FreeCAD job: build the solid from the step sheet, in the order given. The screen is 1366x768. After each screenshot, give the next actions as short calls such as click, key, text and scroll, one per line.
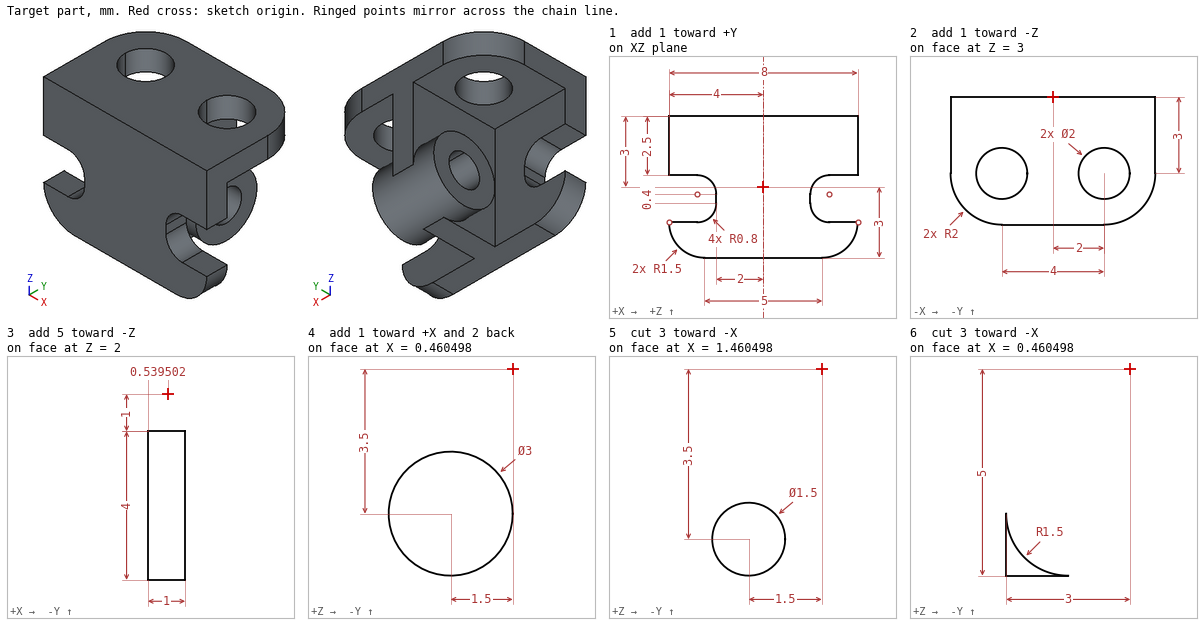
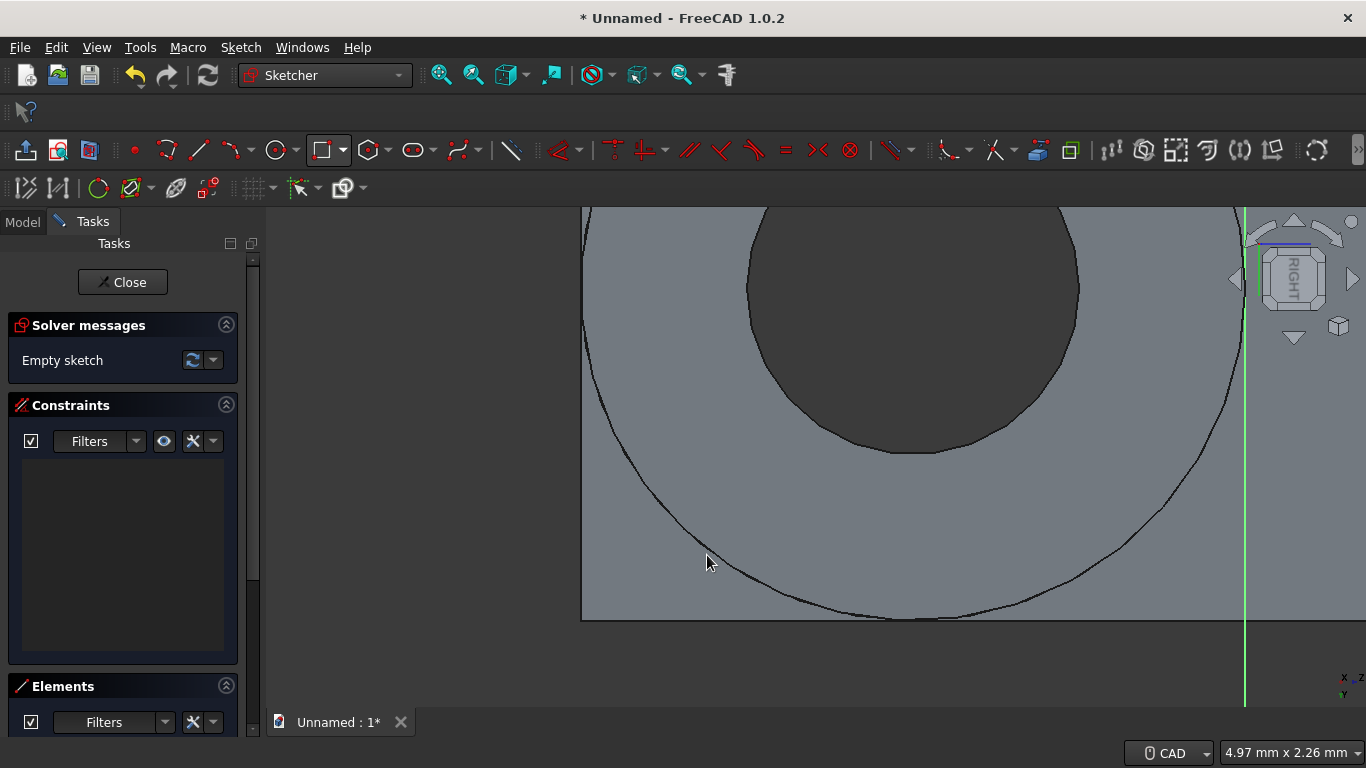
click(168, 150)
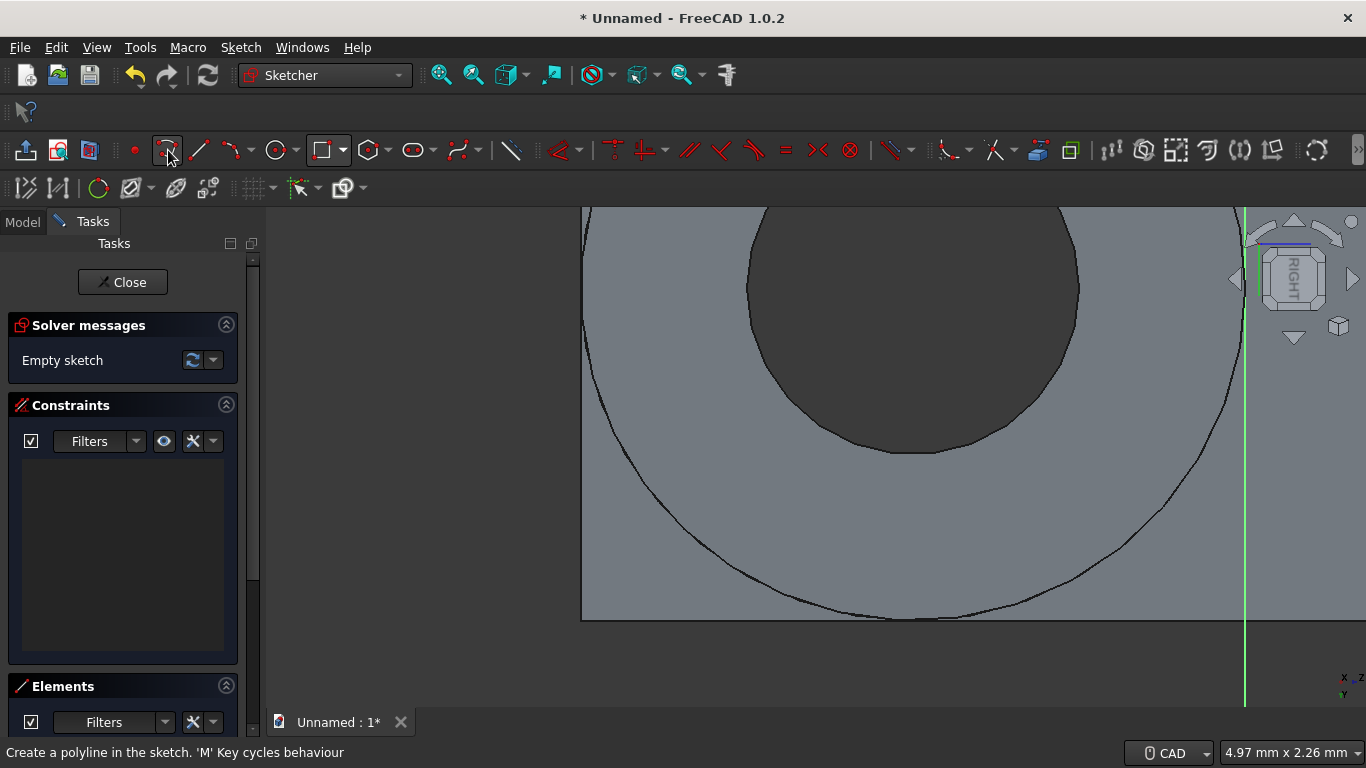
click(581, 288)
click(581, 621)
click(913, 621)
right_click(913, 621)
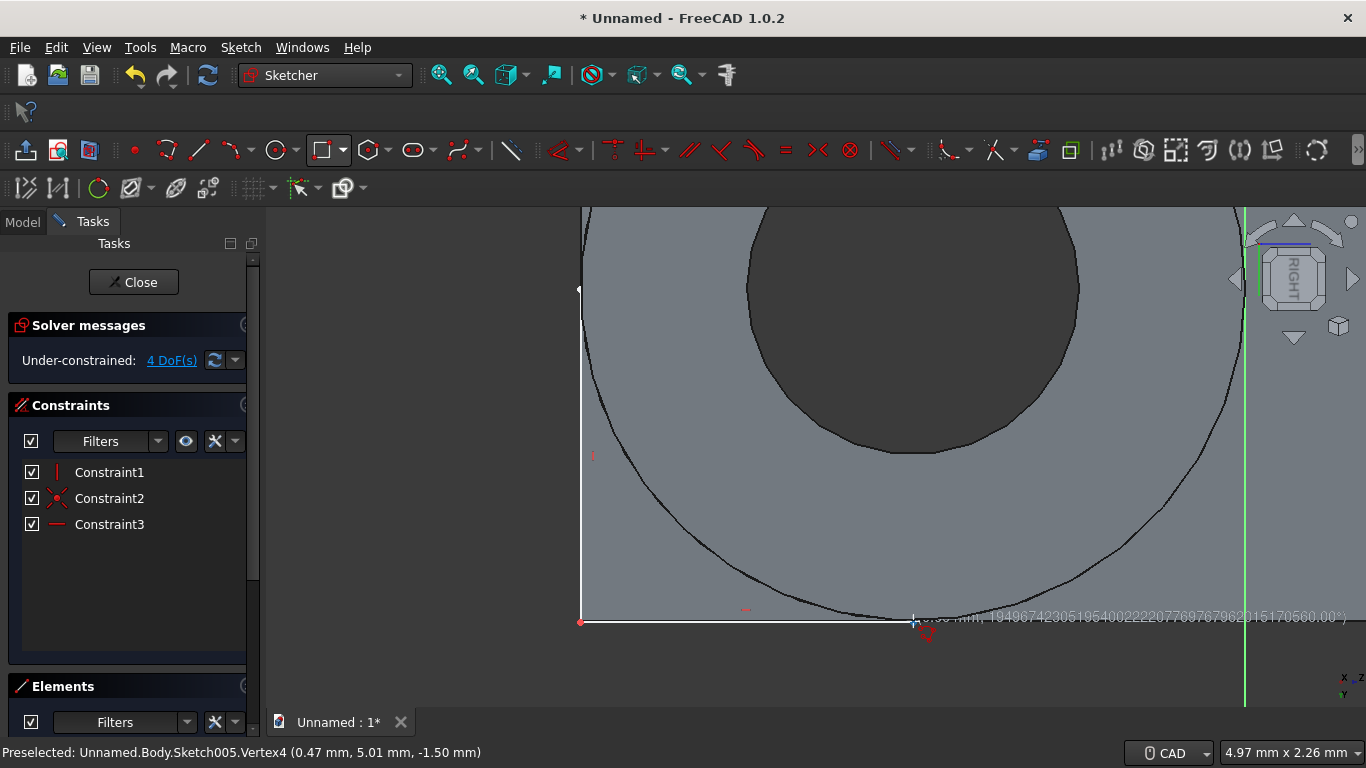
click(232, 150)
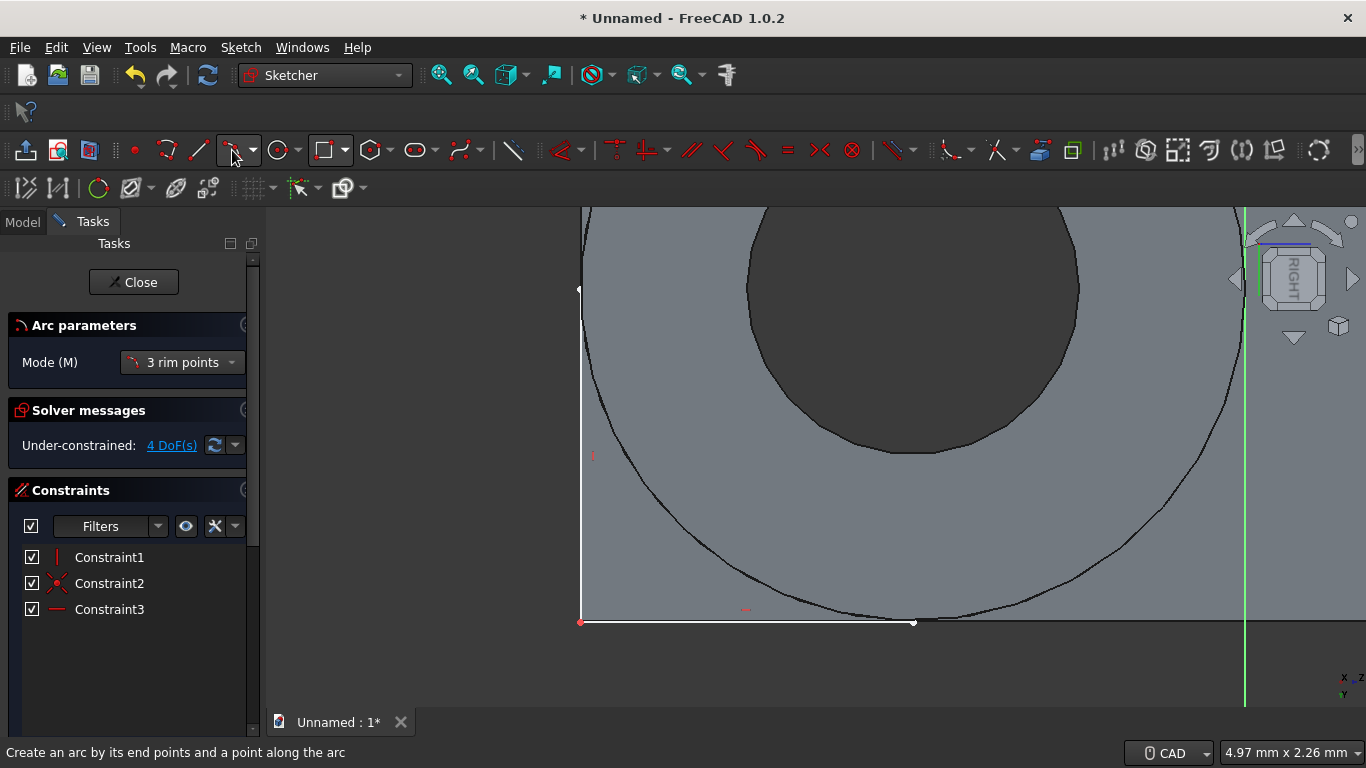
click(913, 622)
click(581, 289)
click(678, 523)
key(Escape)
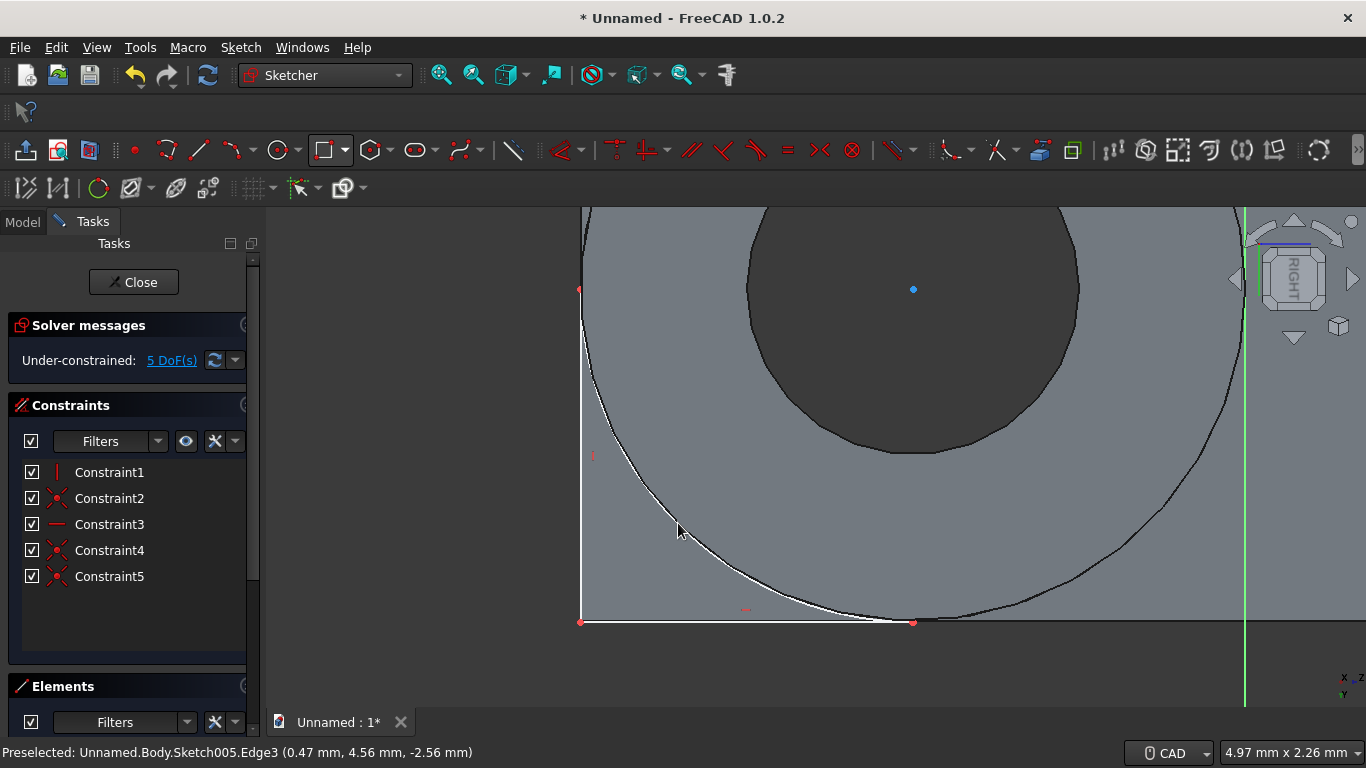
click(581, 389)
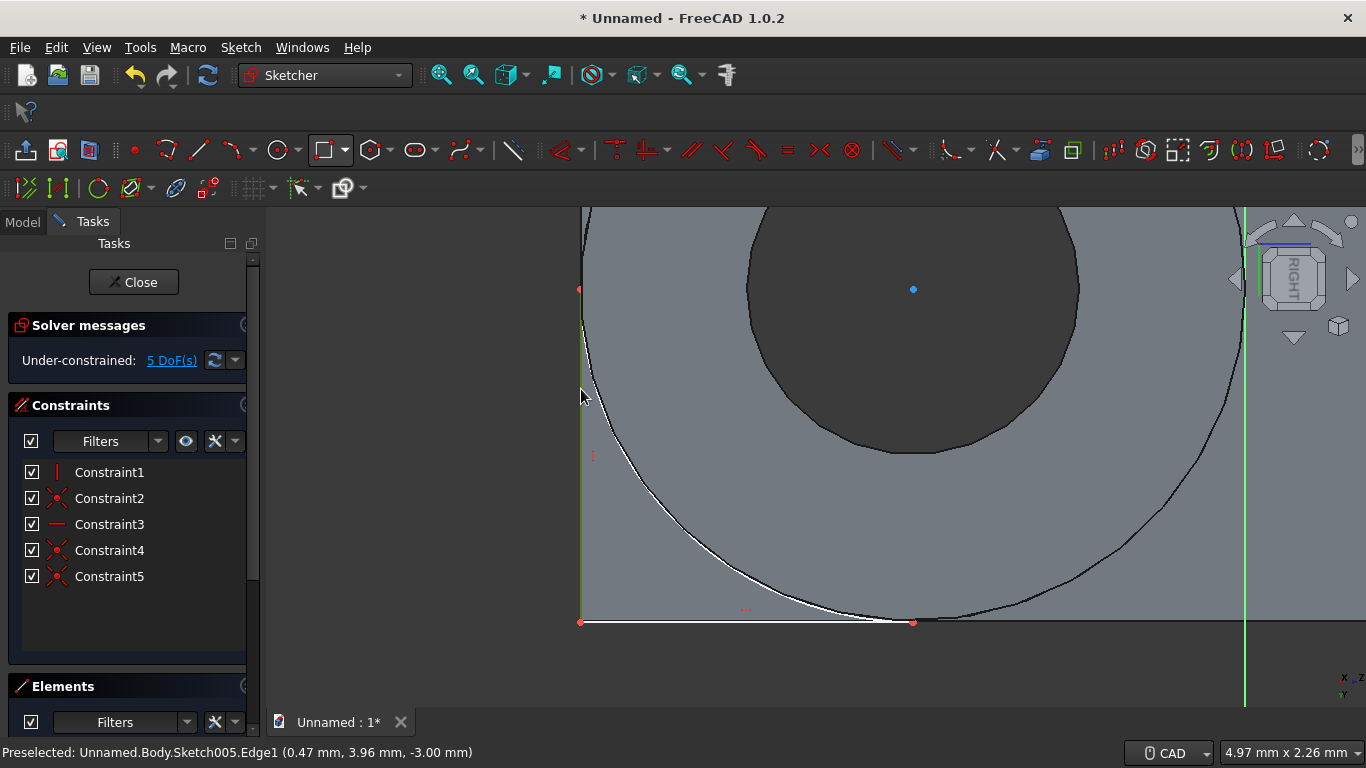
click(617, 440)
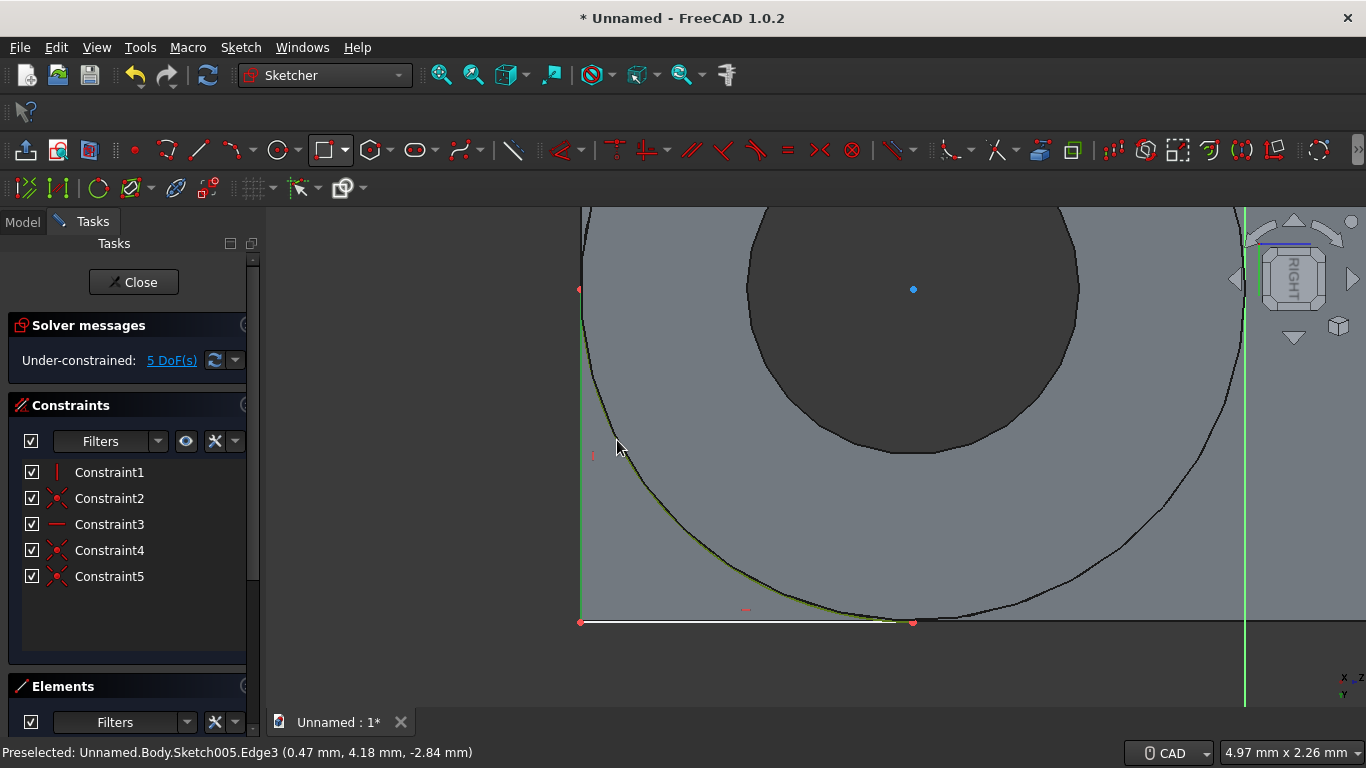
click(756, 150)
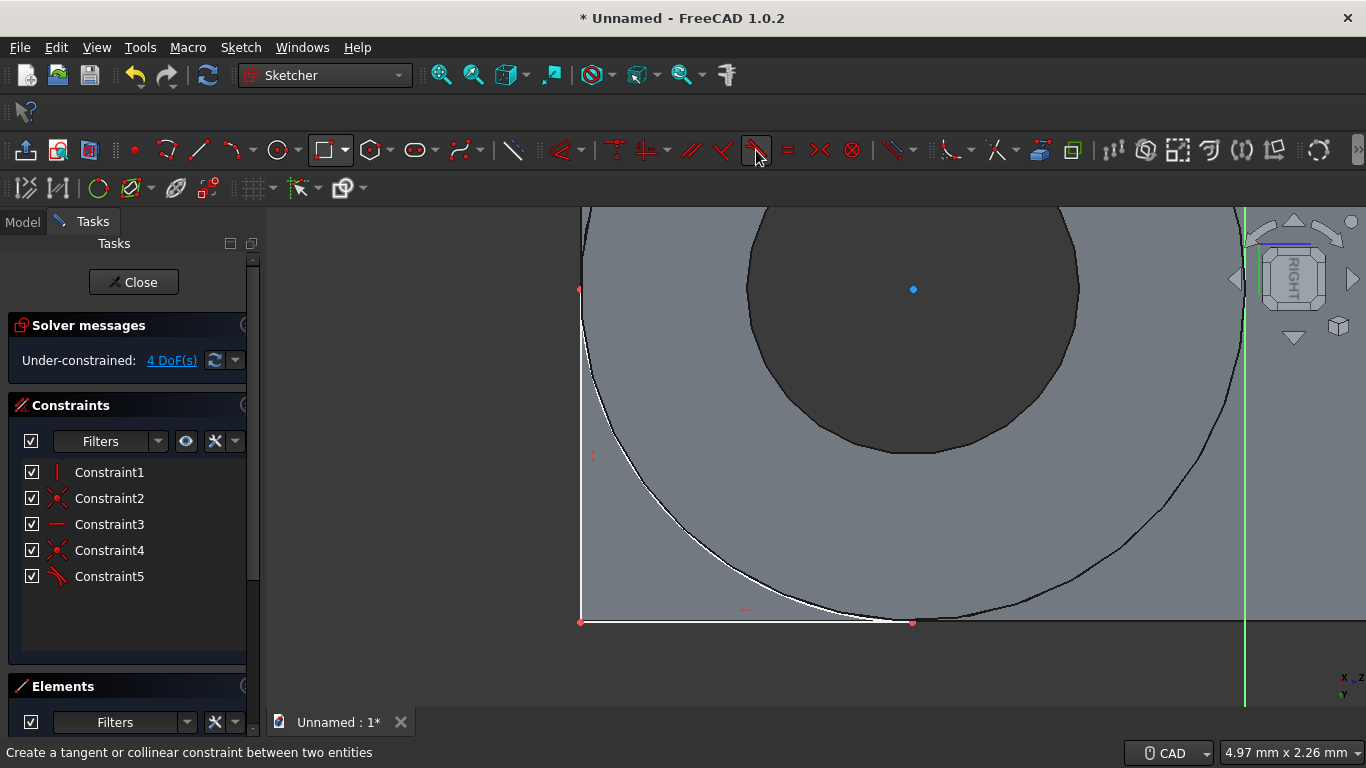
click(681, 622)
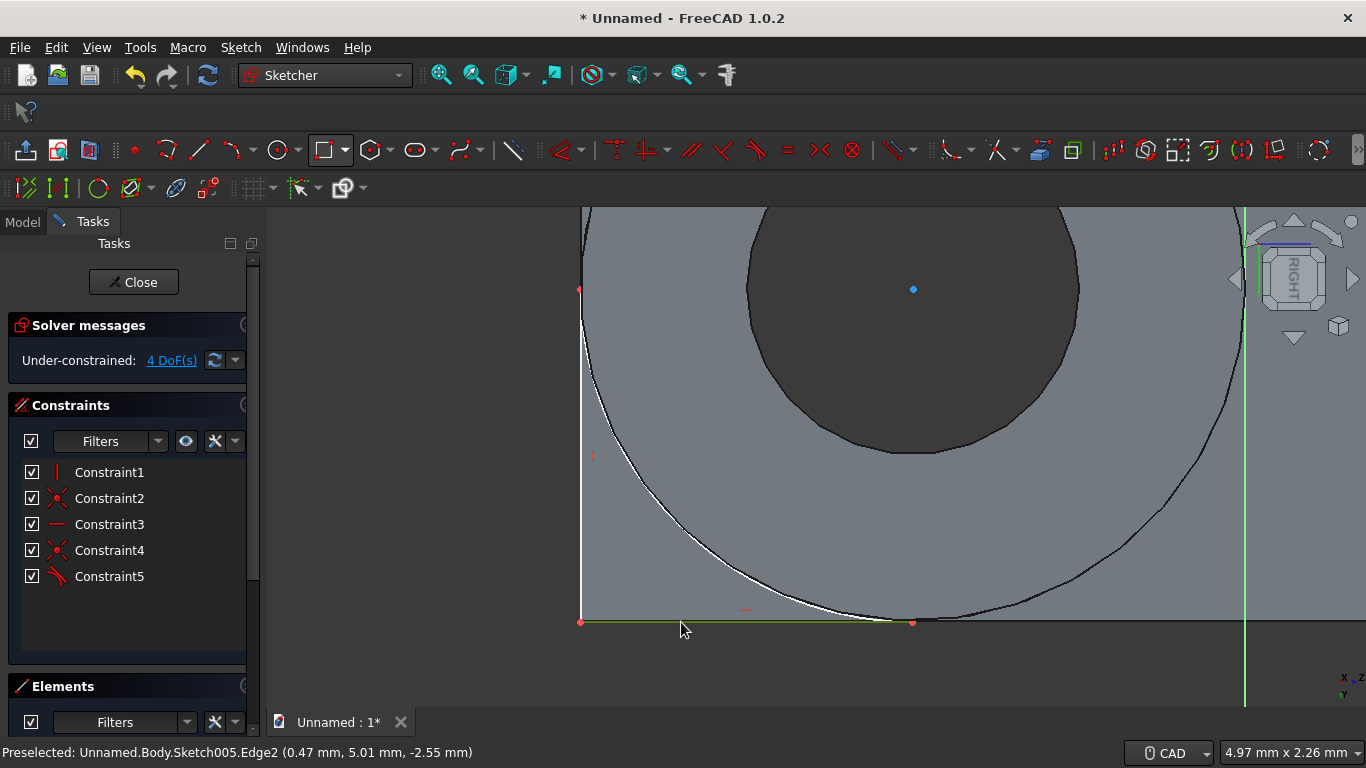
click(617, 440)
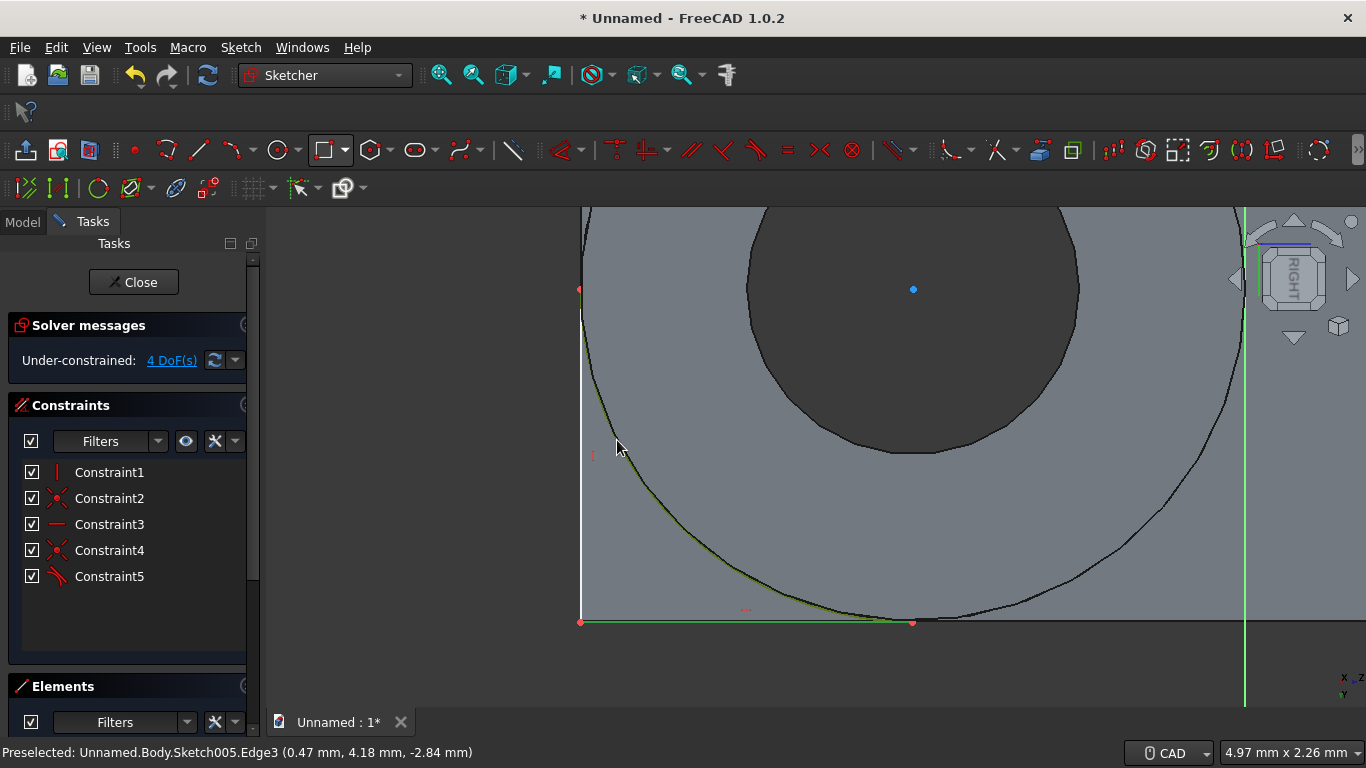
click(756, 150)